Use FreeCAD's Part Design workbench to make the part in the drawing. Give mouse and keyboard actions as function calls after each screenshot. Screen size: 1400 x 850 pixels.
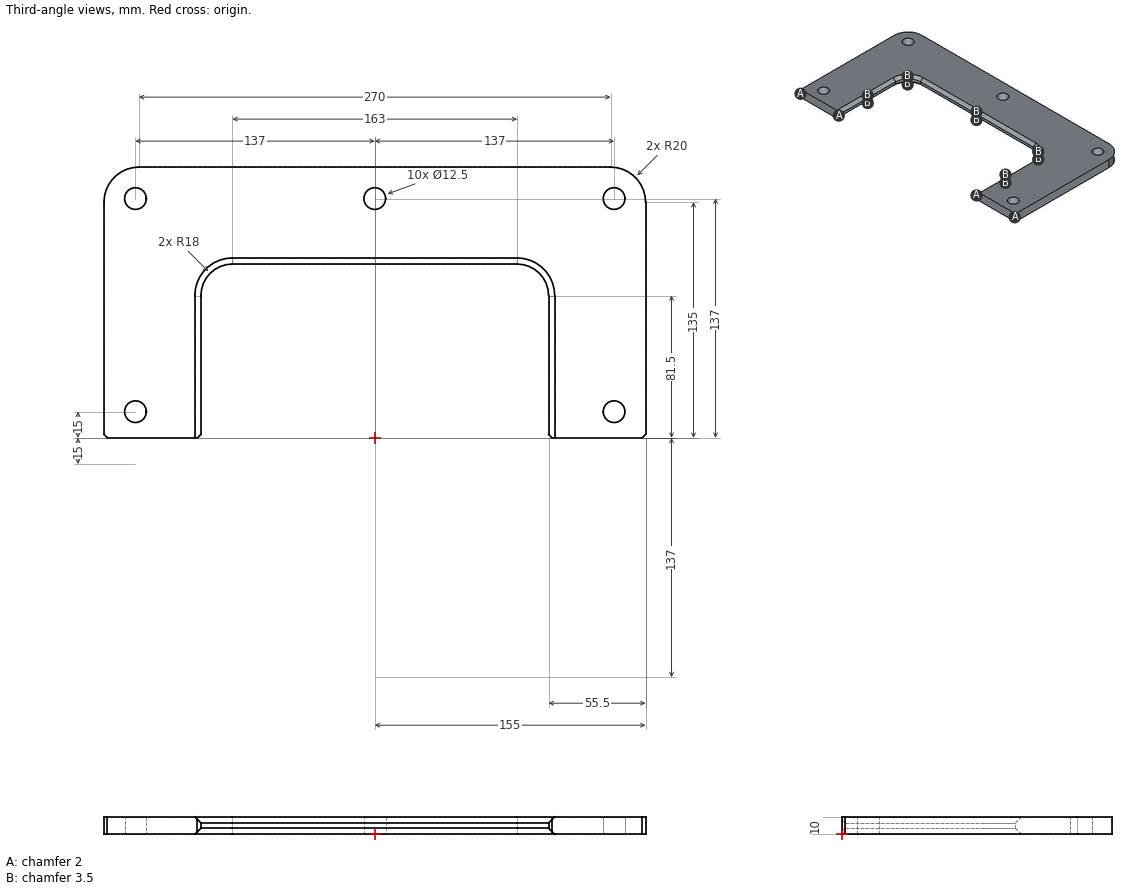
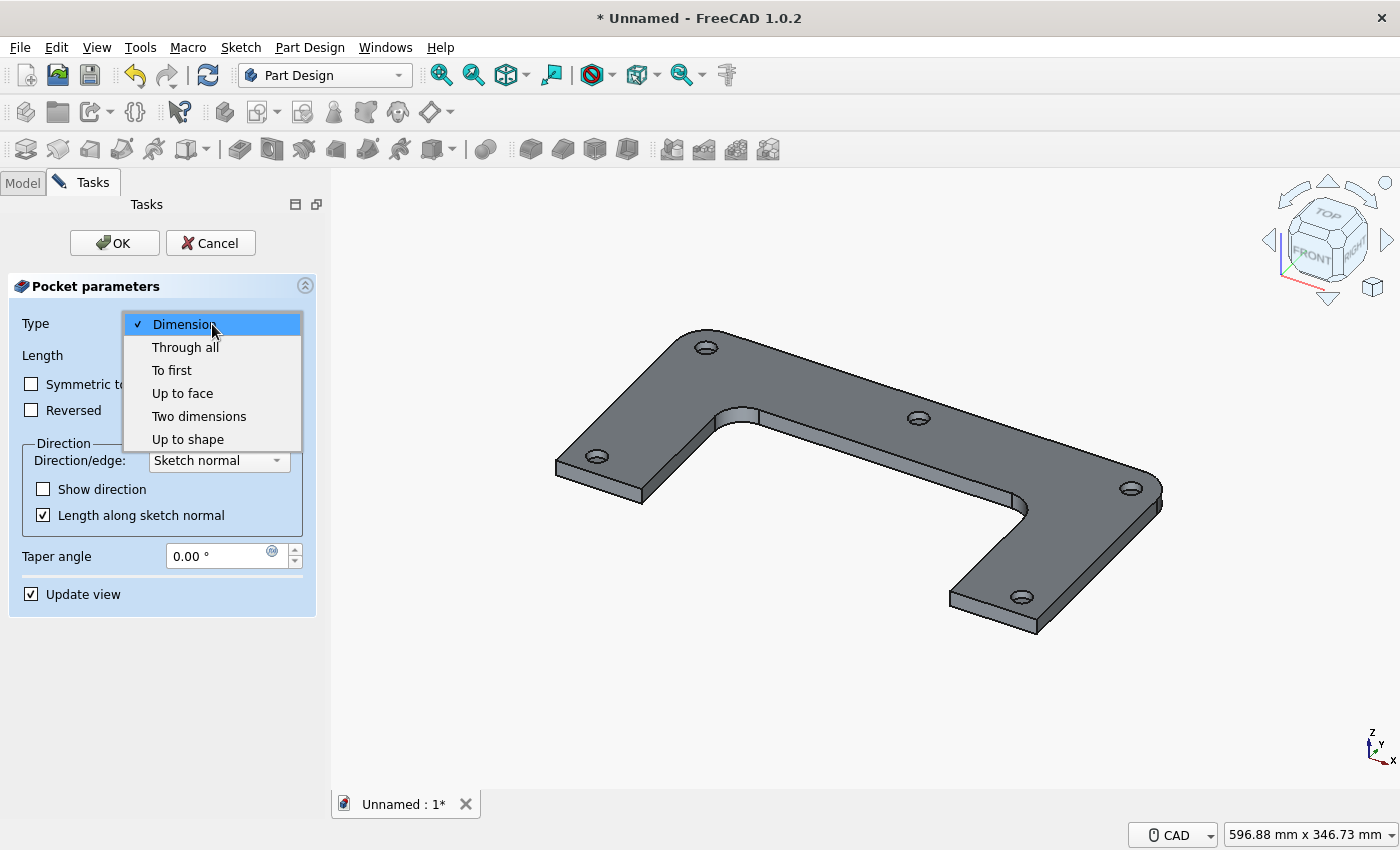
click(212, 348)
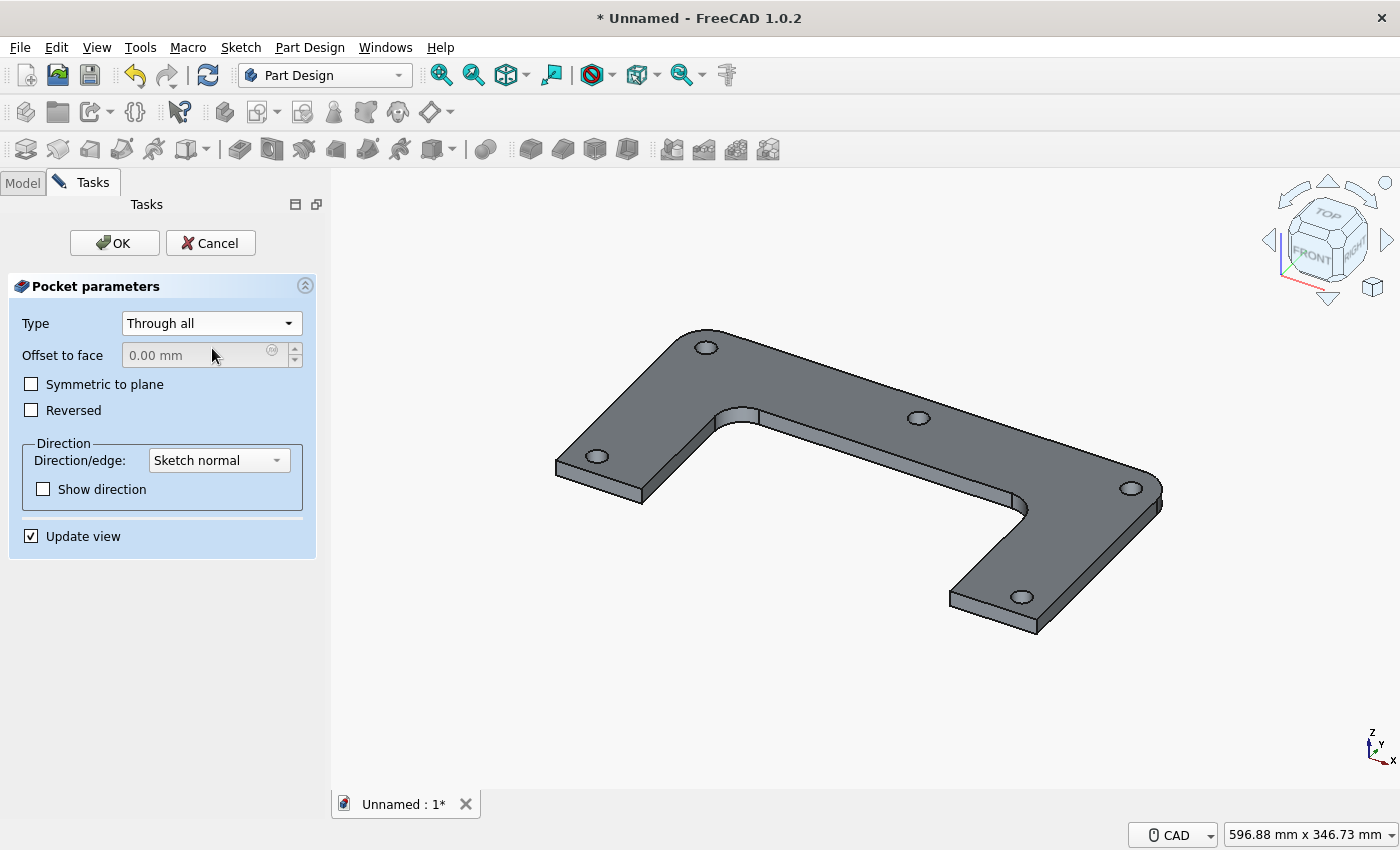
click(115, 243)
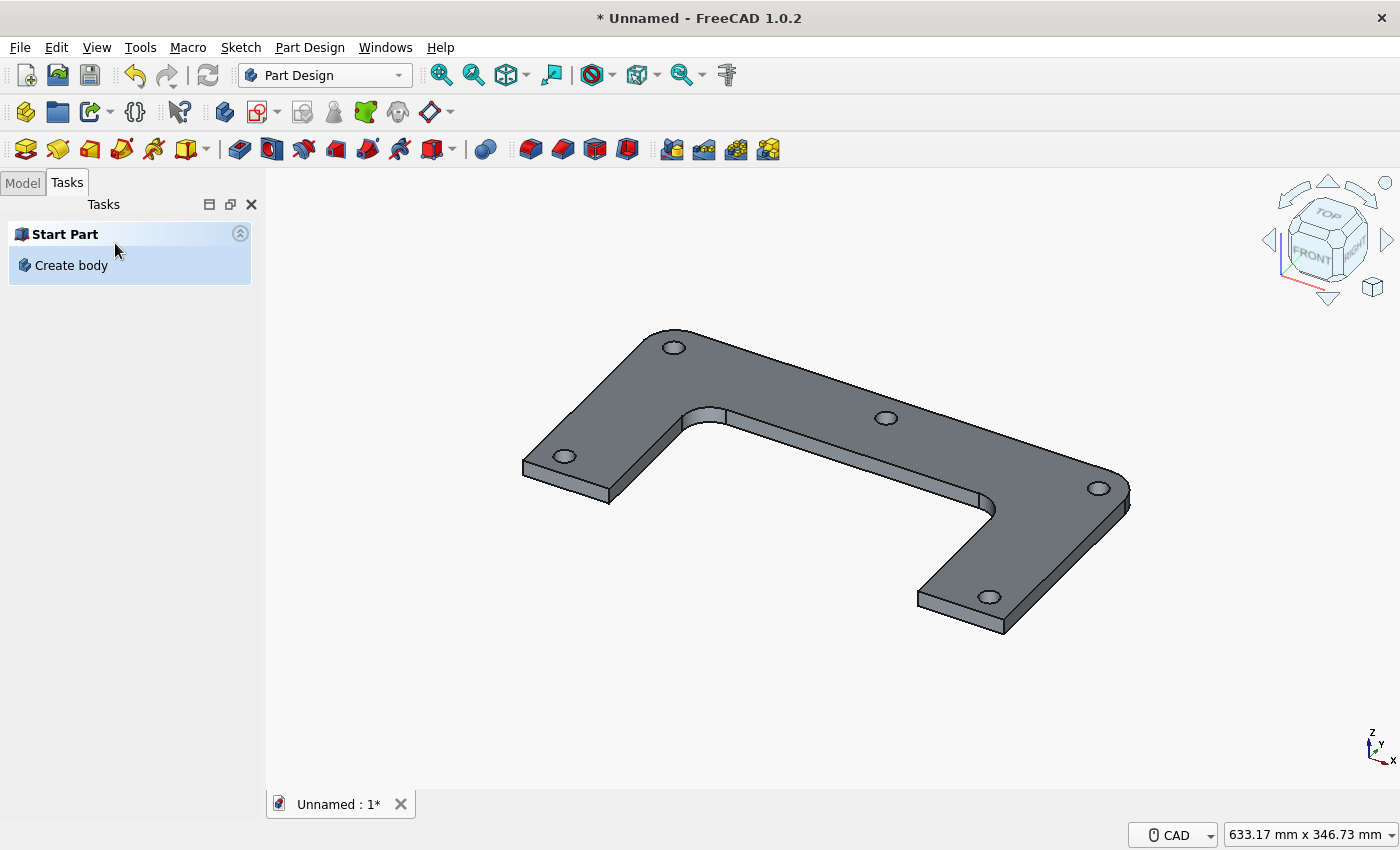
click(609, 495)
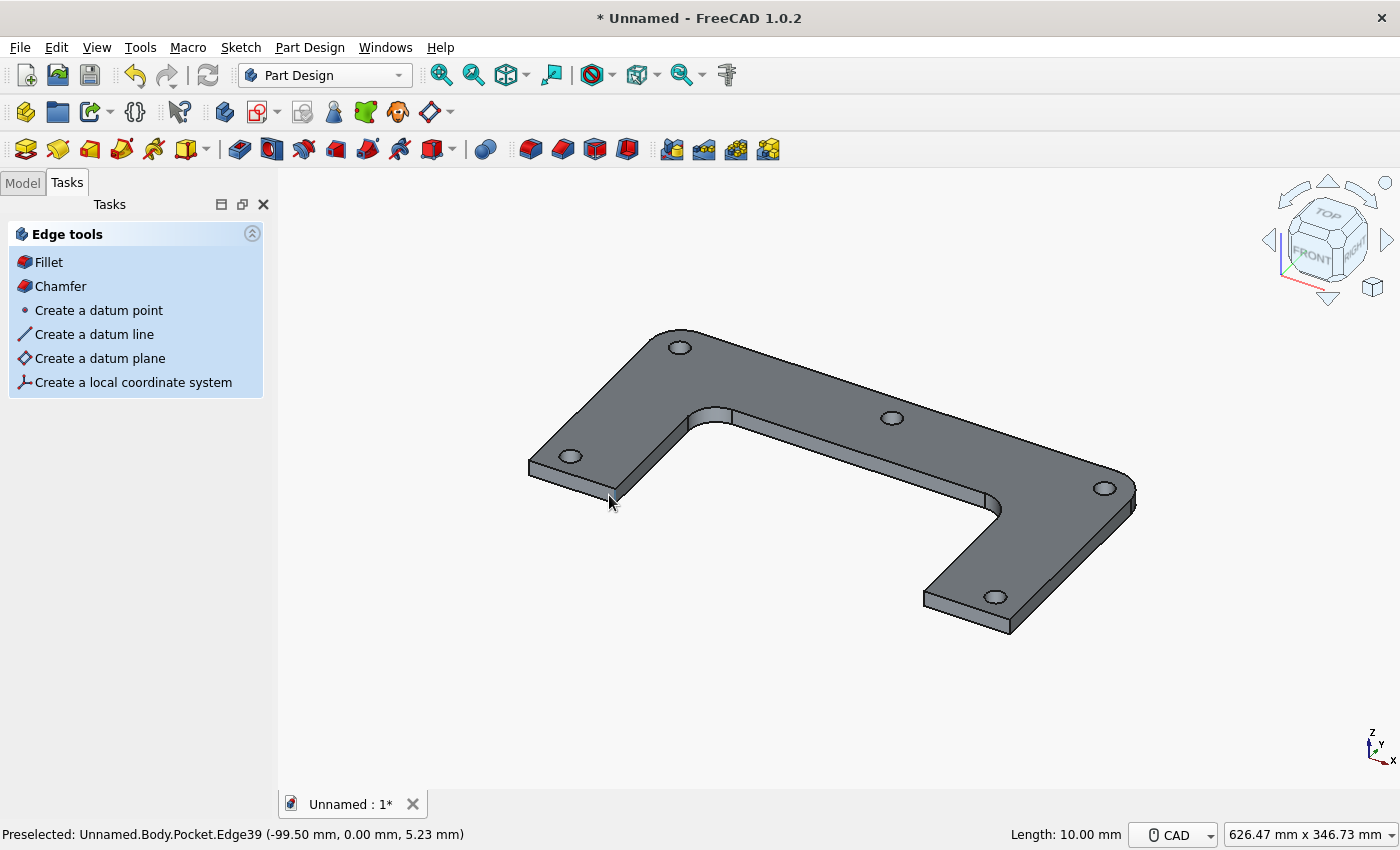
click(1010, 626, ctrl)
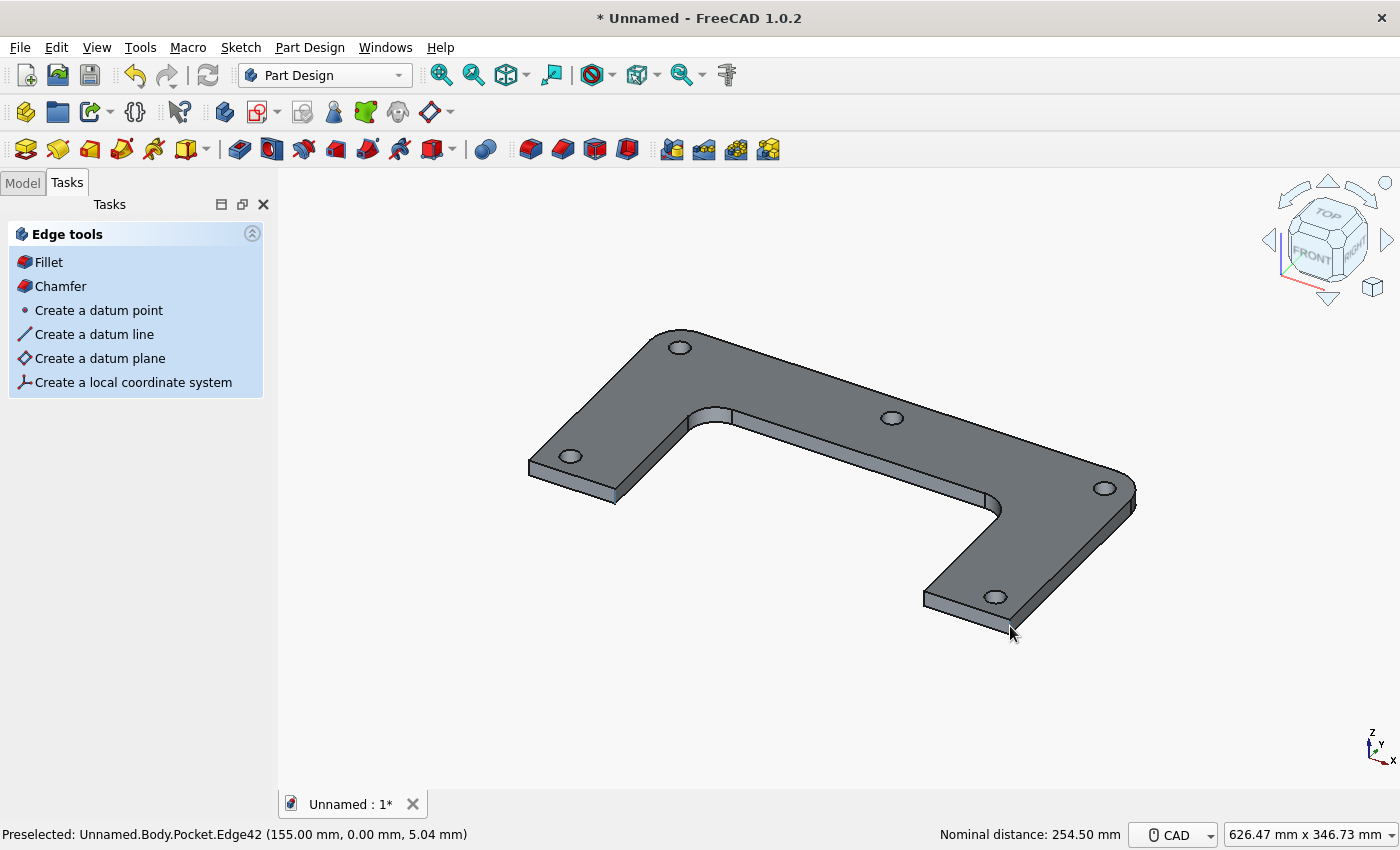
scroll(529, 467, up, 5)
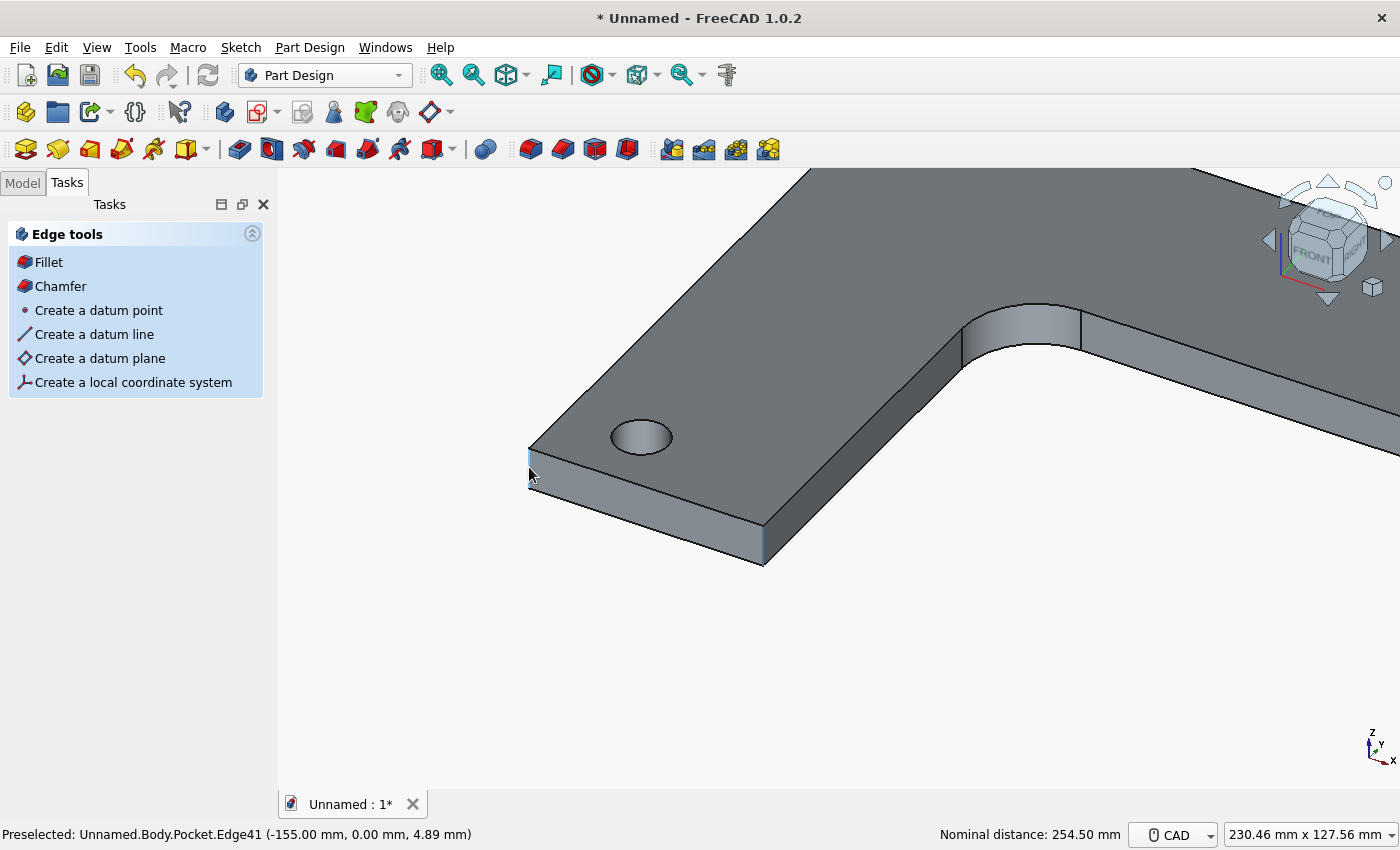
key(v)
key(f)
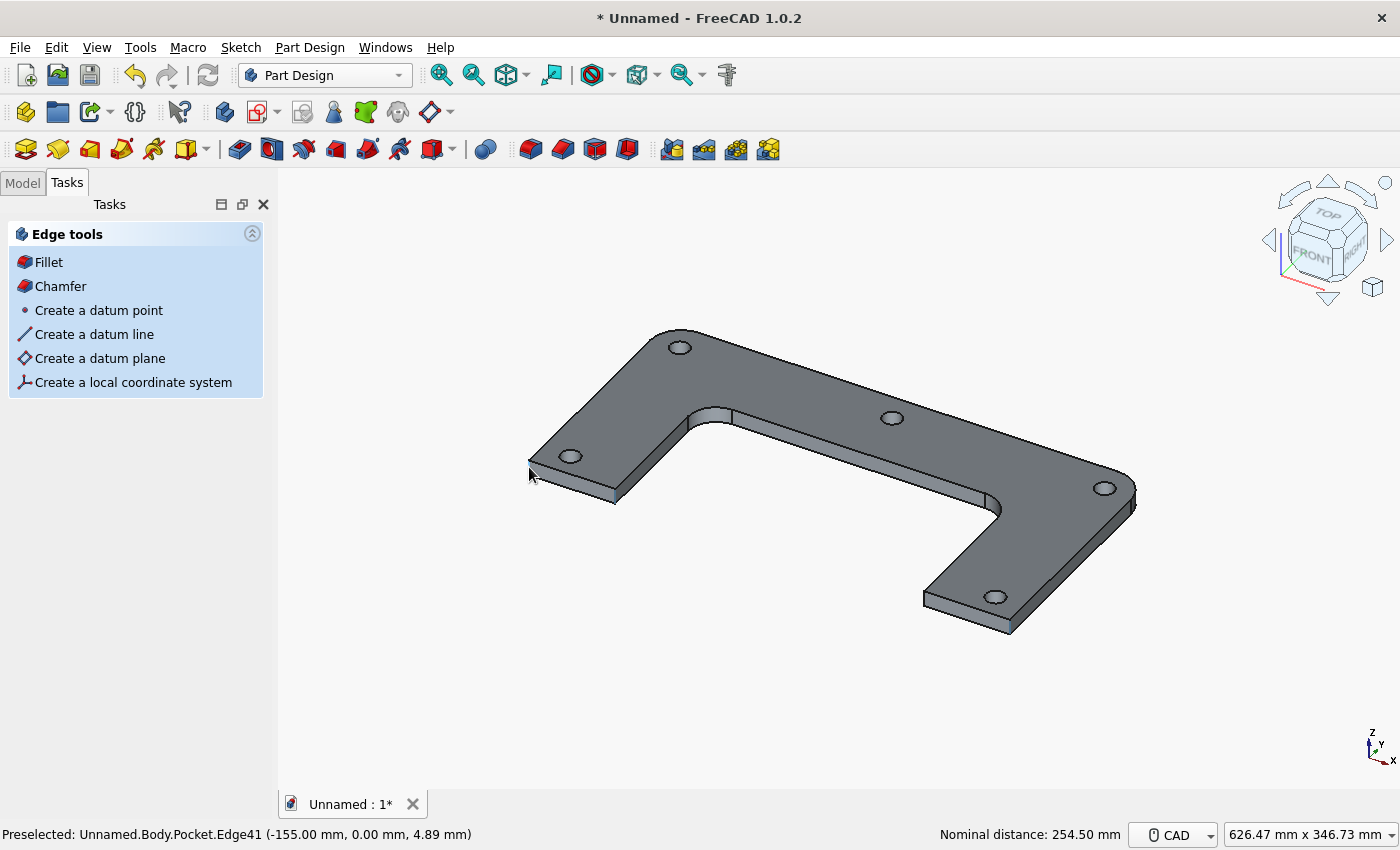
key(0)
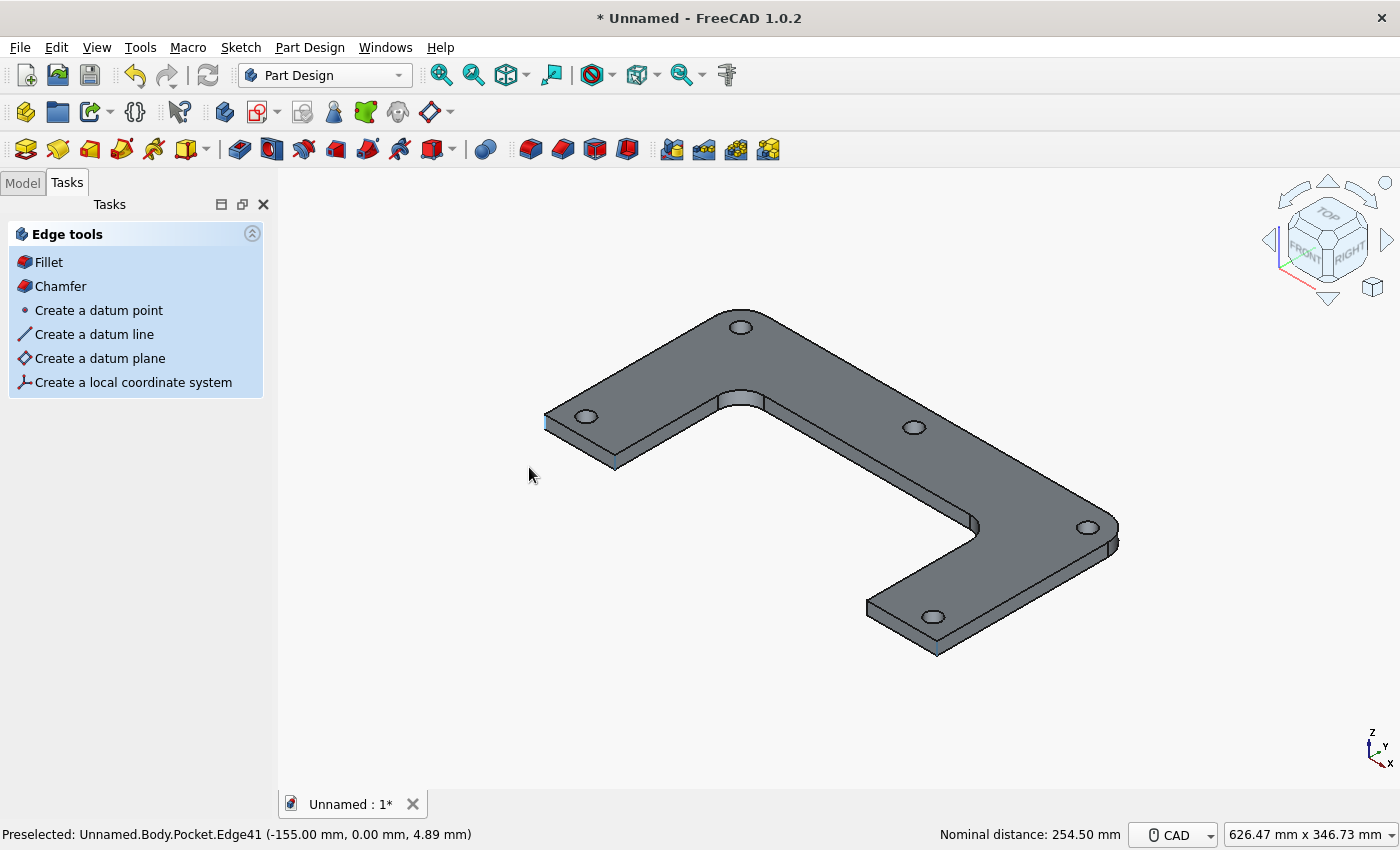
scroll(545, 421, up, 5)